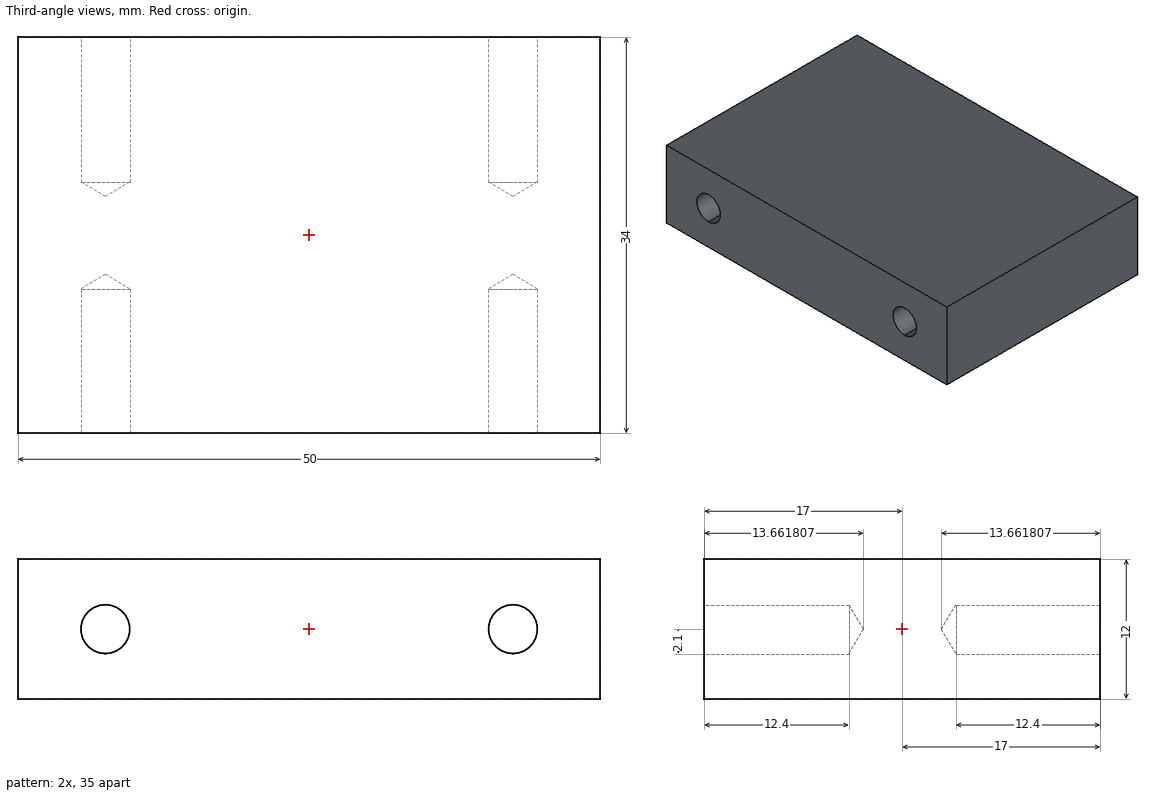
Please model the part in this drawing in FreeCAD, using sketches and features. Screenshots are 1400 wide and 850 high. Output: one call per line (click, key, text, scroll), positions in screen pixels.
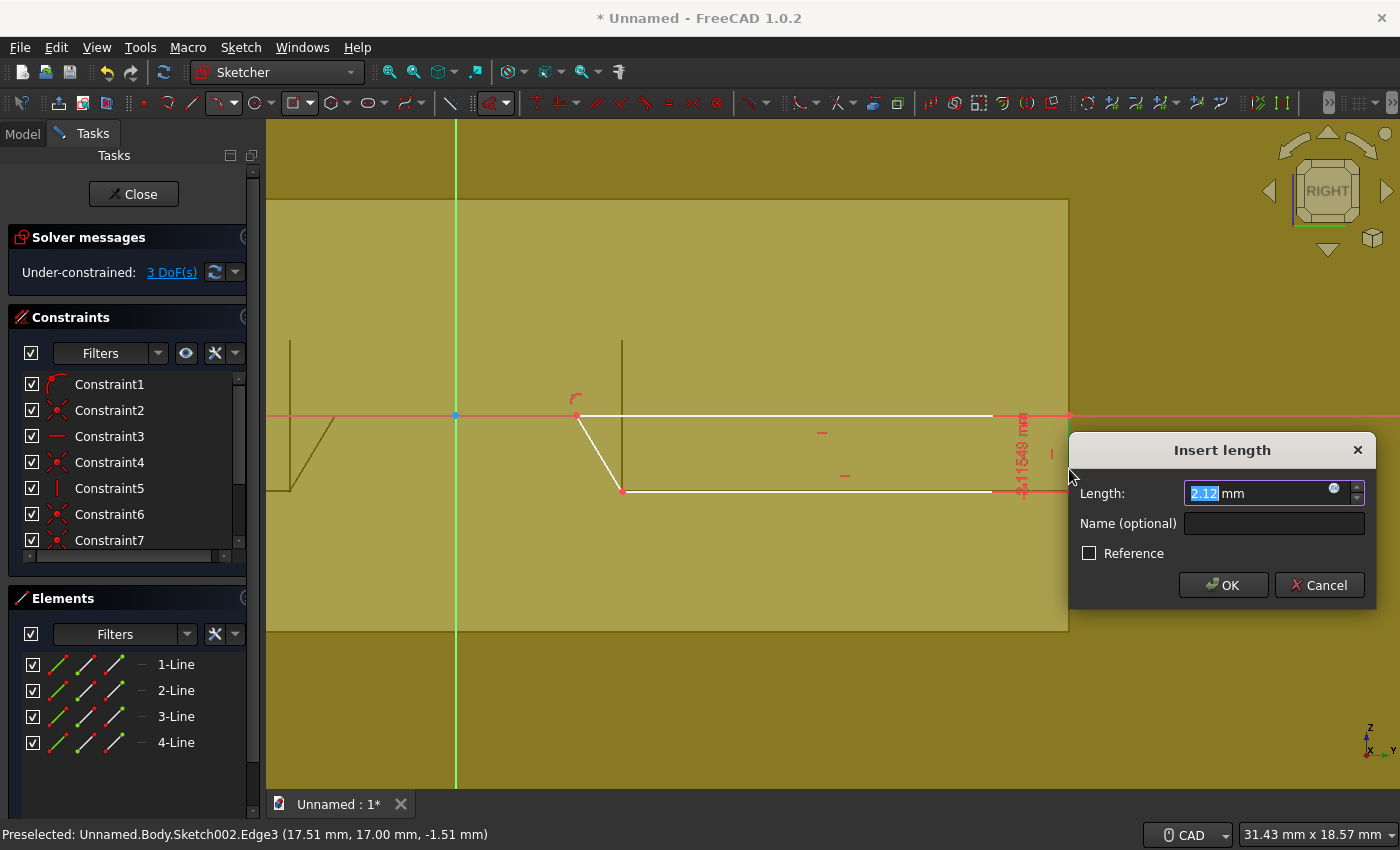
text(2.1)
key(Return)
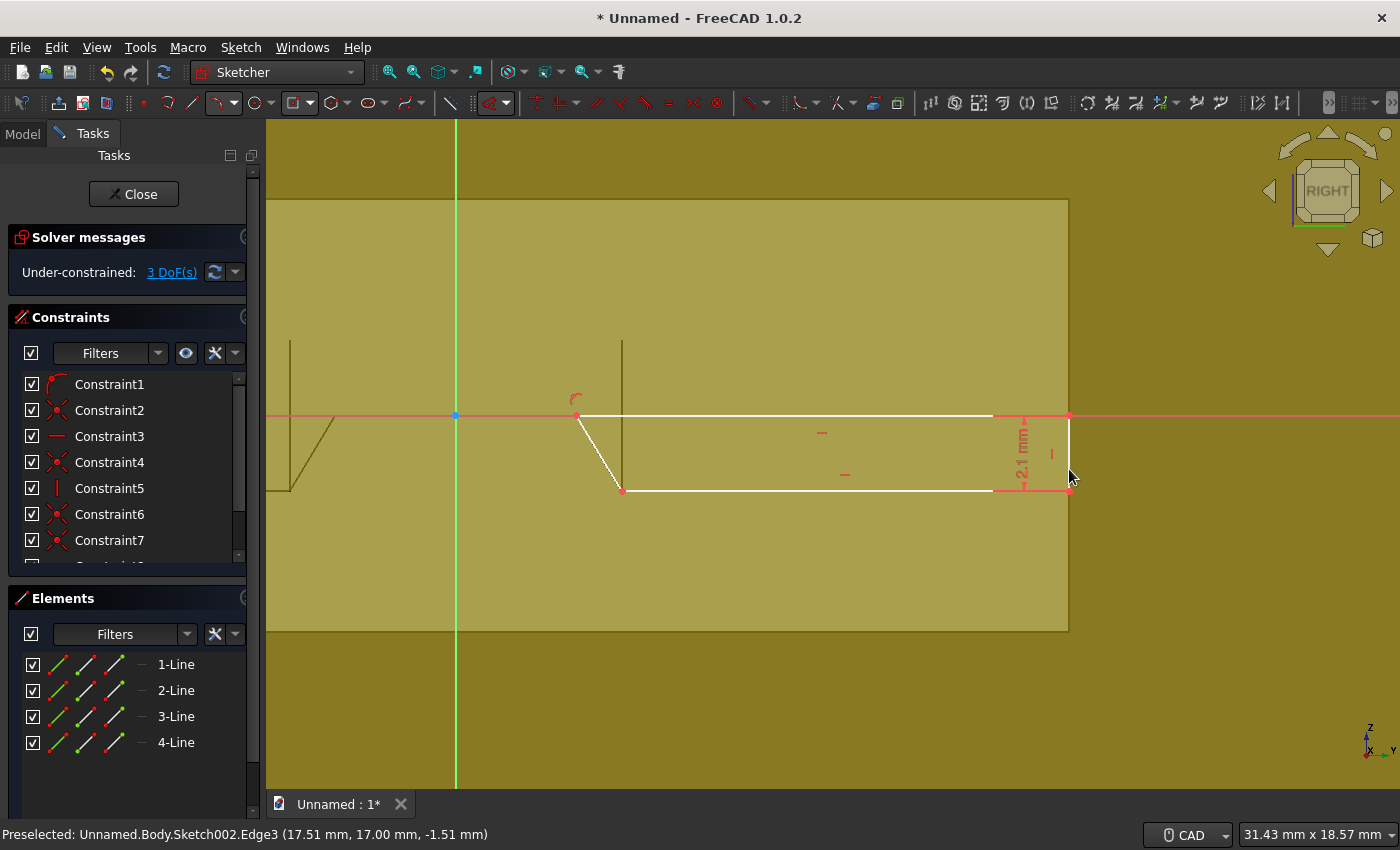
click(1069, 491)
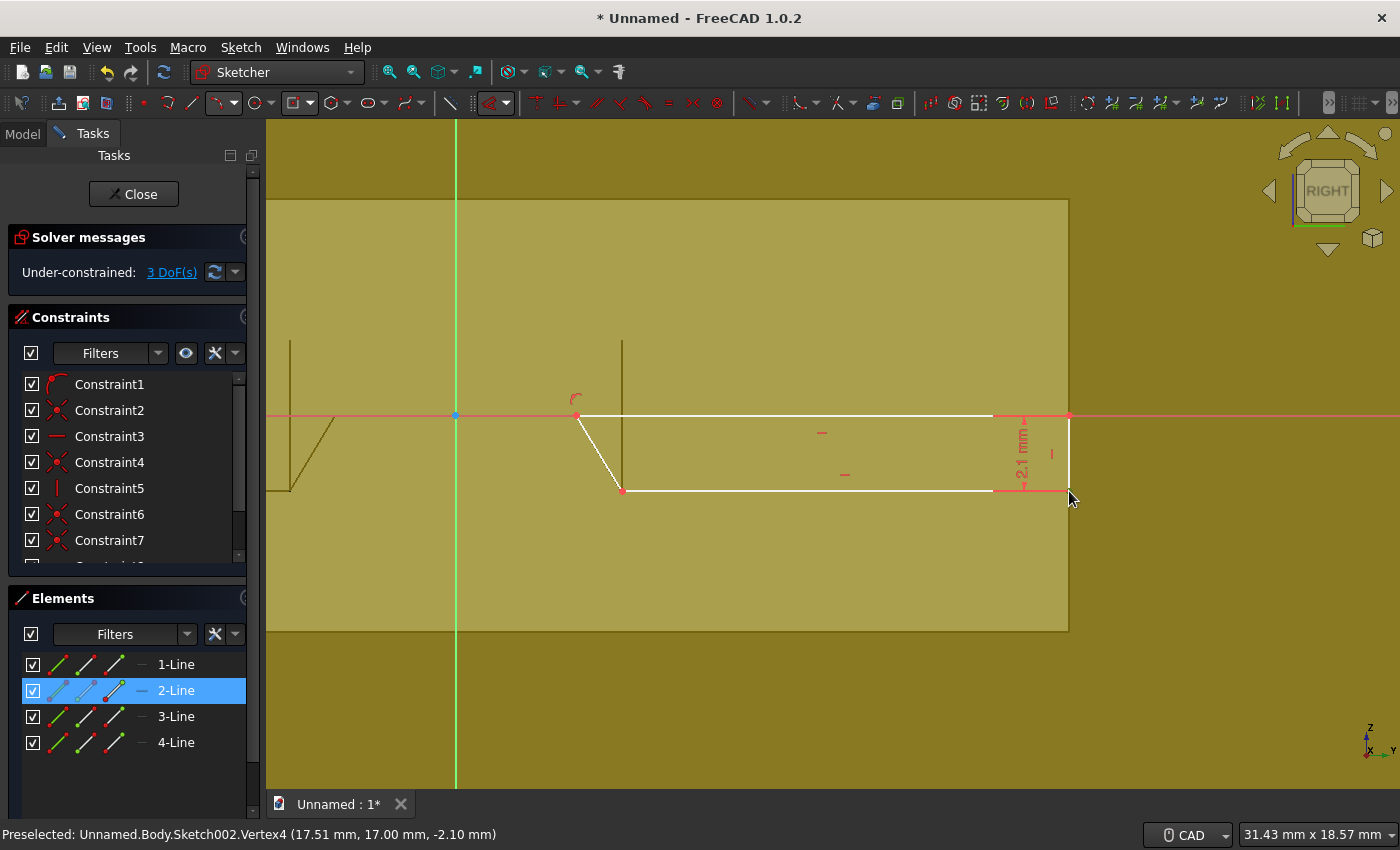
click(508, 104)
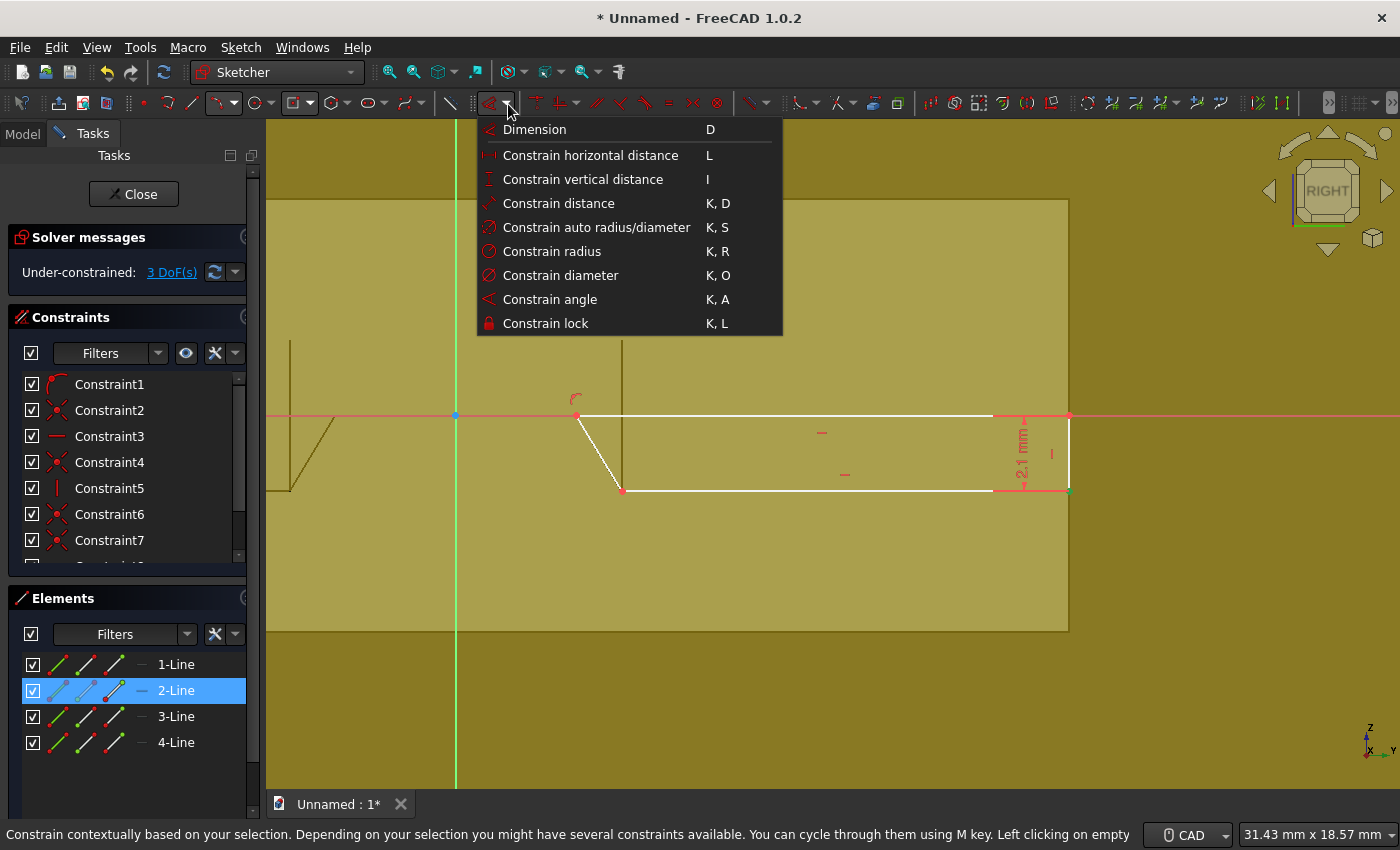
click(630, 155)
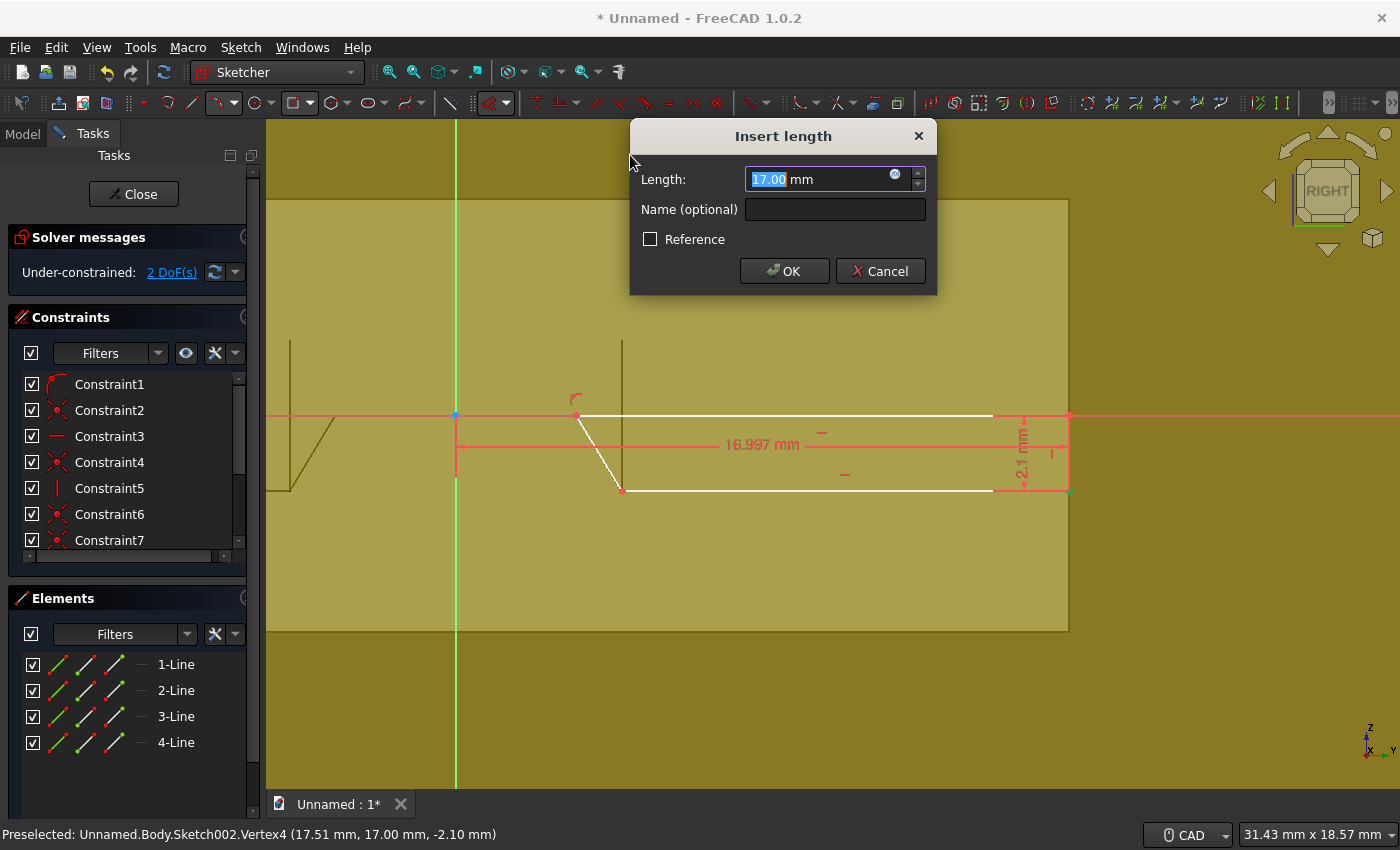
text(17)
key(Return)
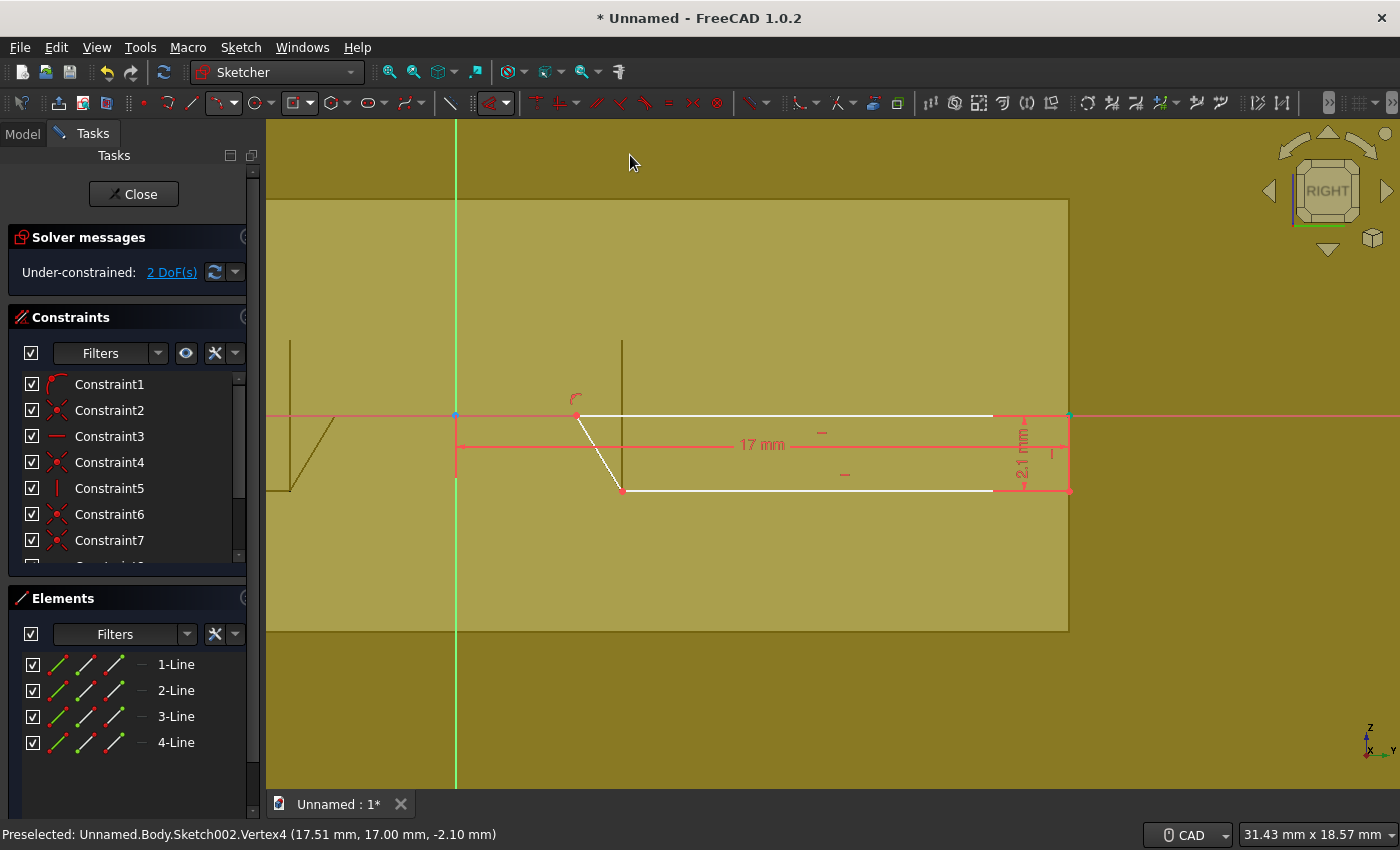
click(756, 491)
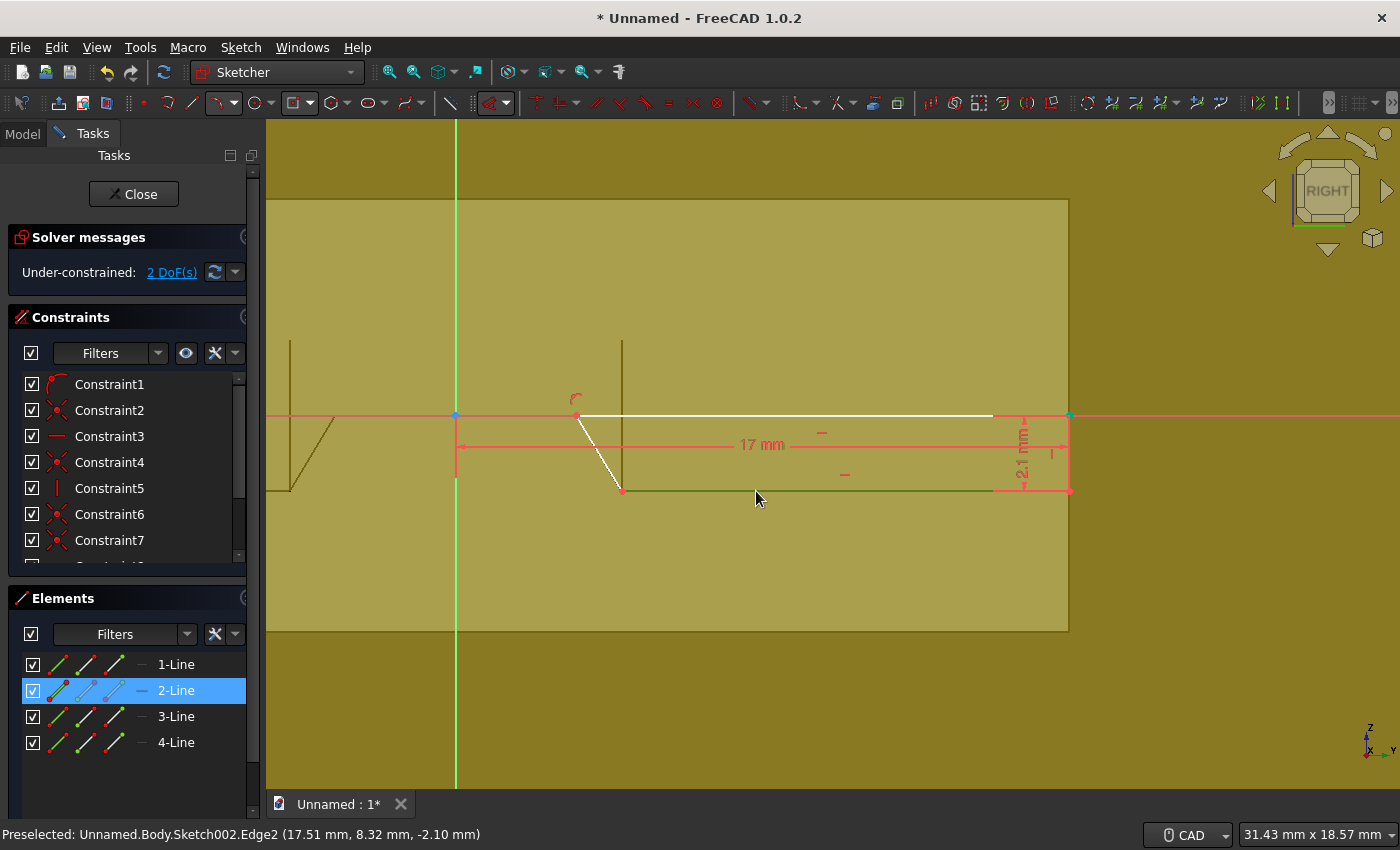
key(l)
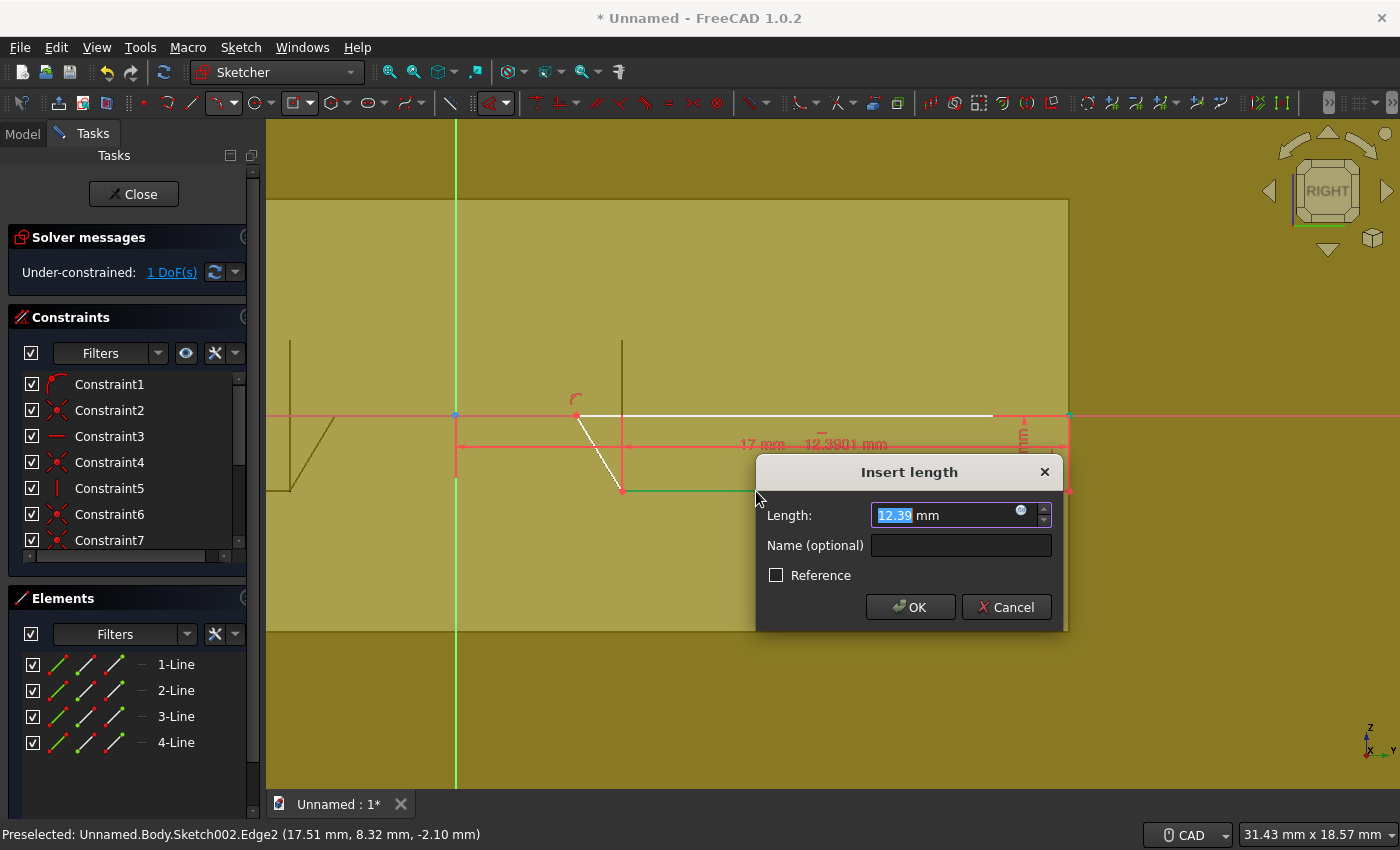
text(12.4)
key(Return)